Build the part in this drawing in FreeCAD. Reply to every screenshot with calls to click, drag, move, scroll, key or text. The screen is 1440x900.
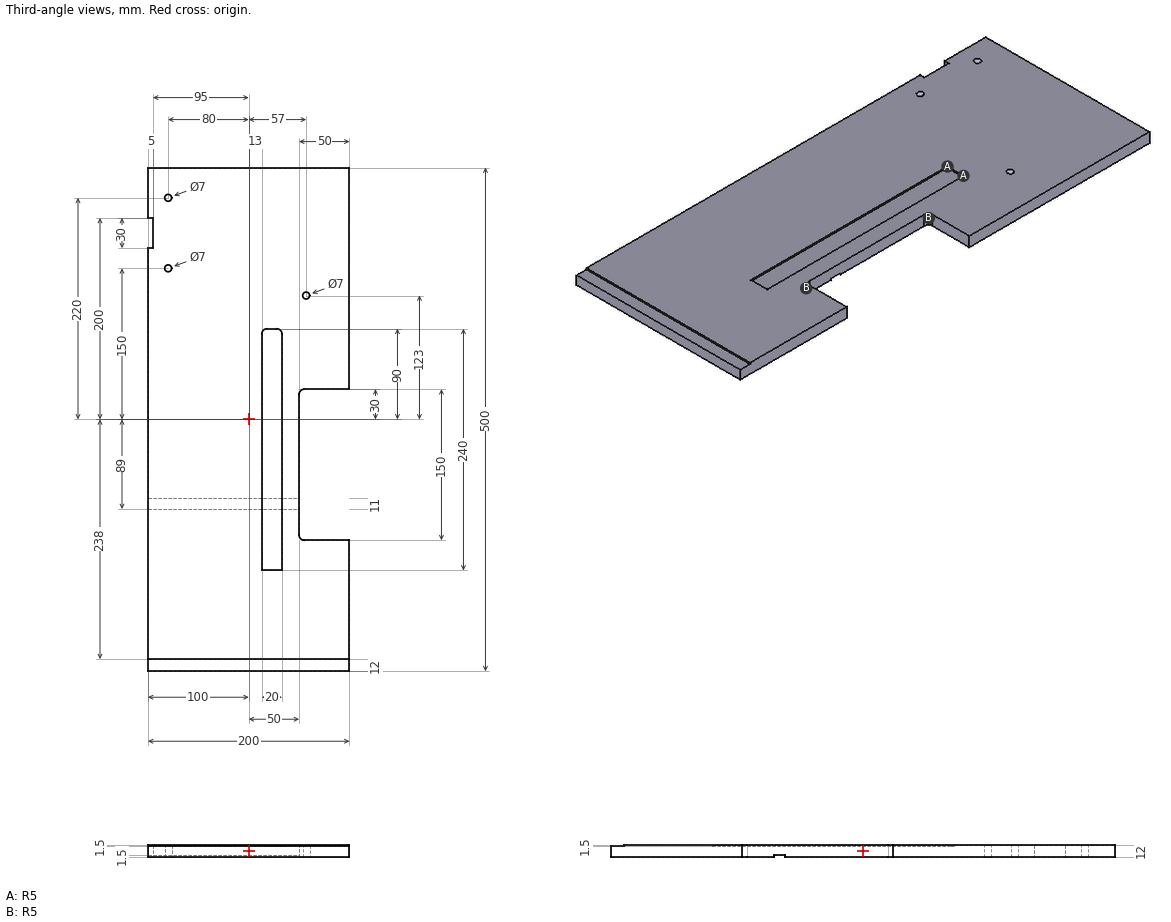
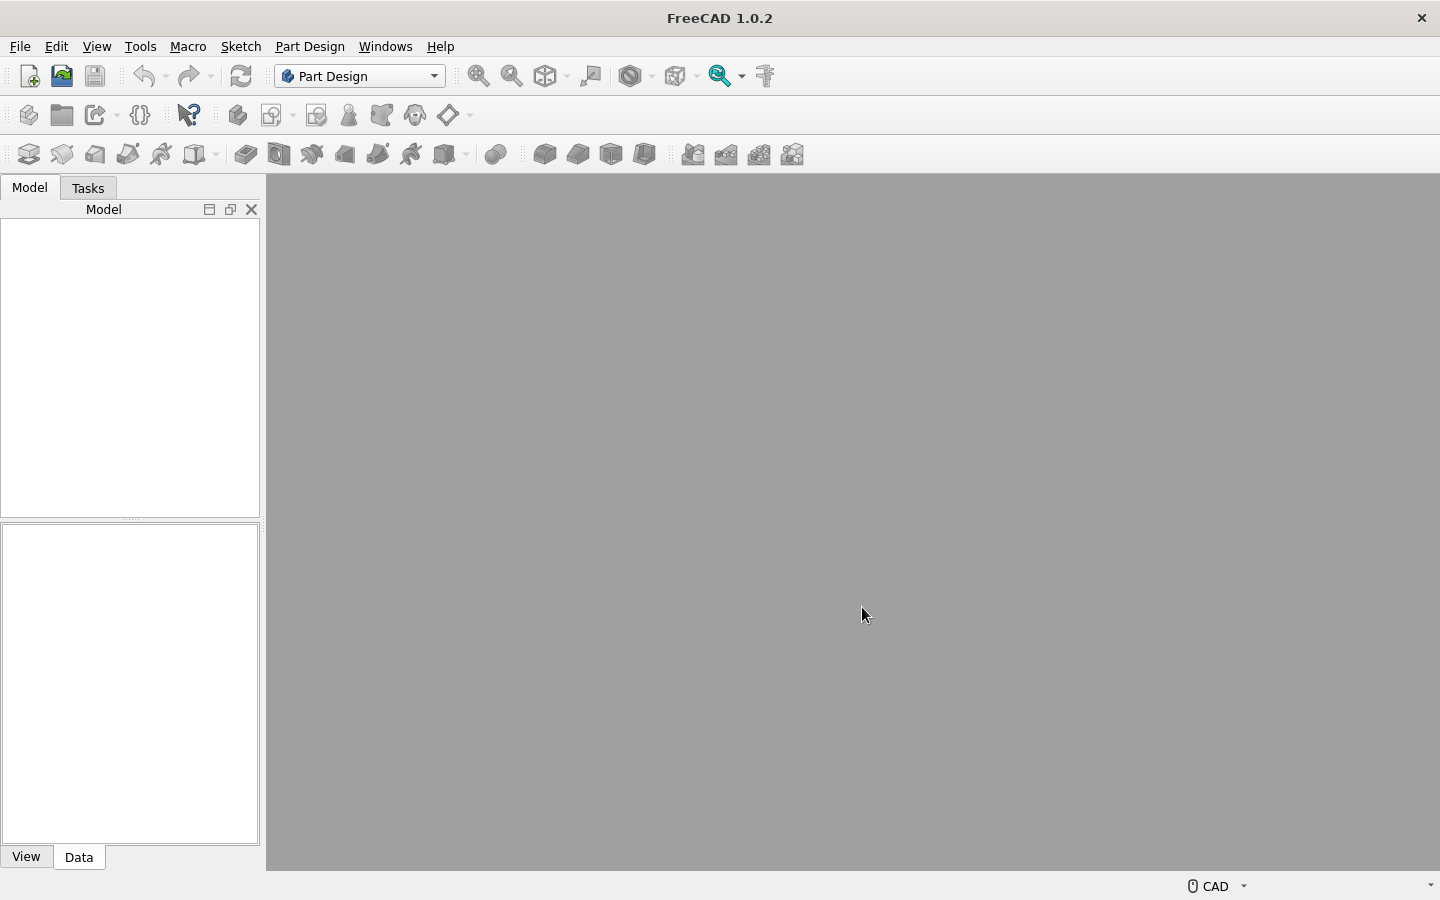
click(29, 76)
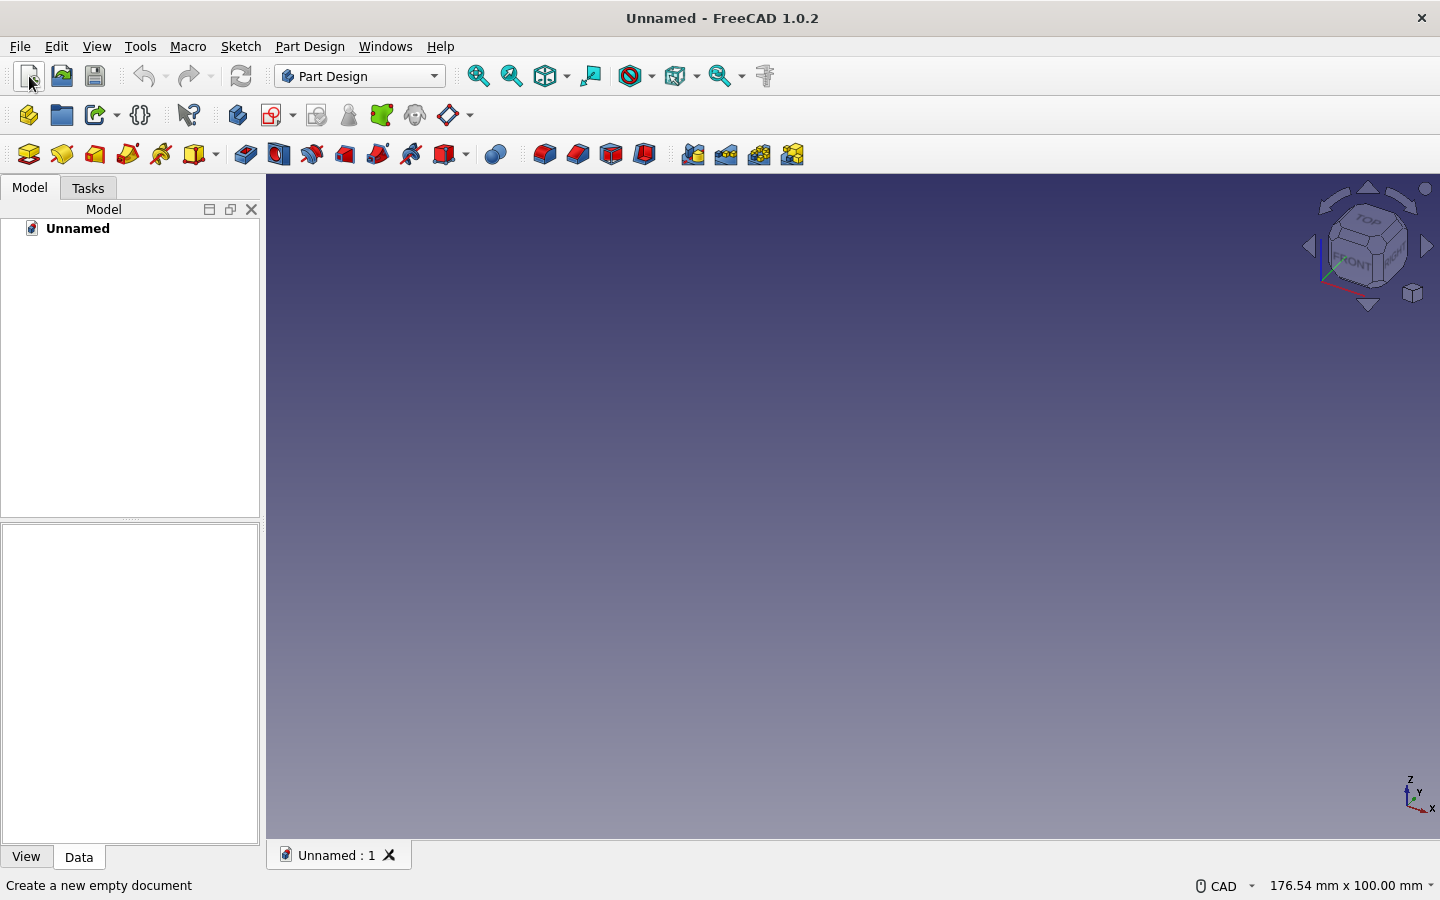
click(270, 116)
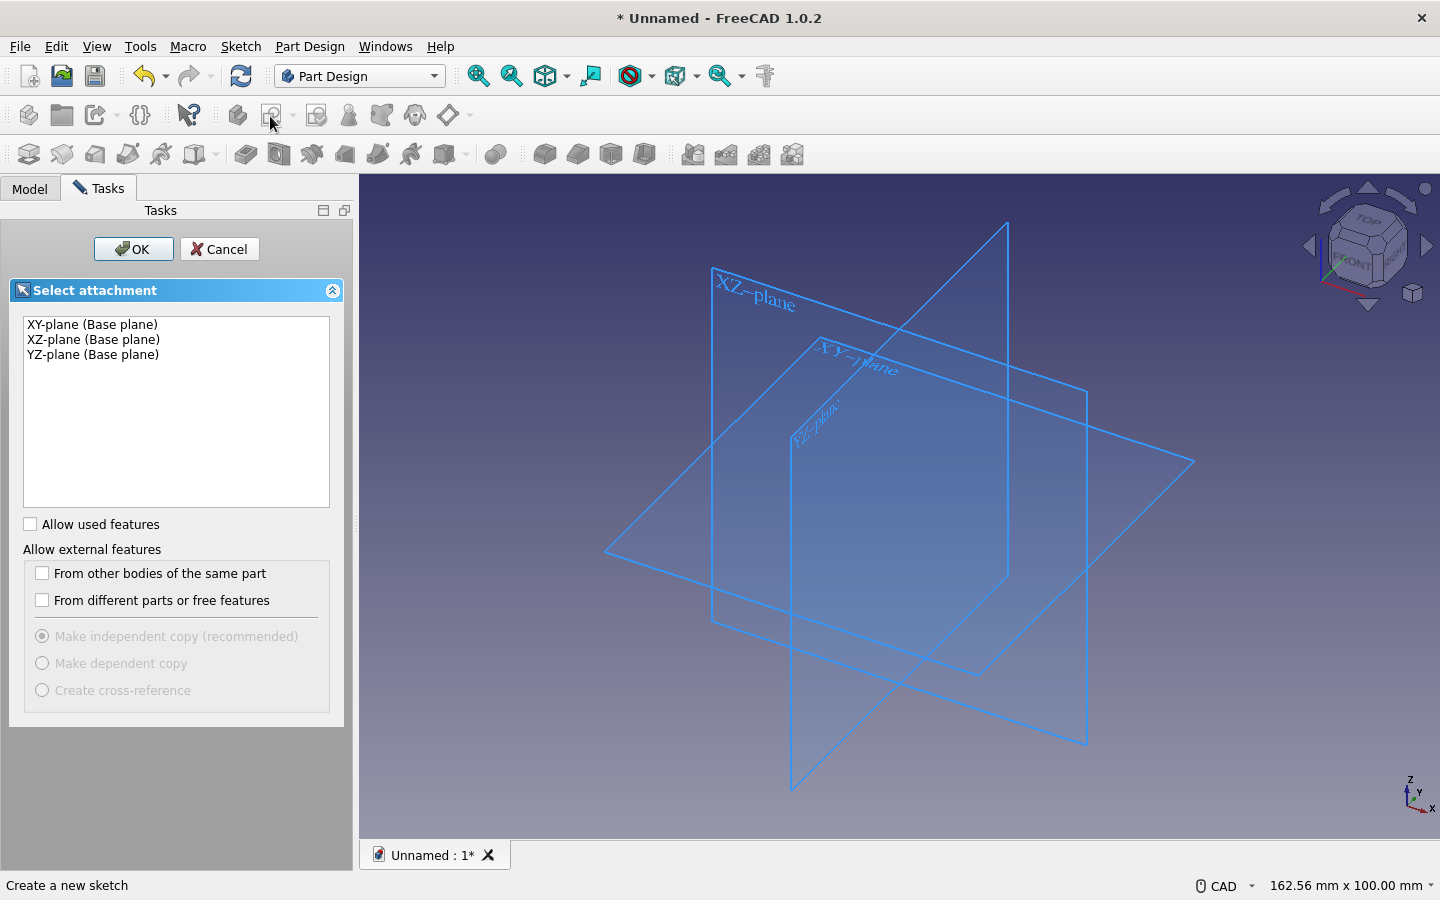
click(84, 324)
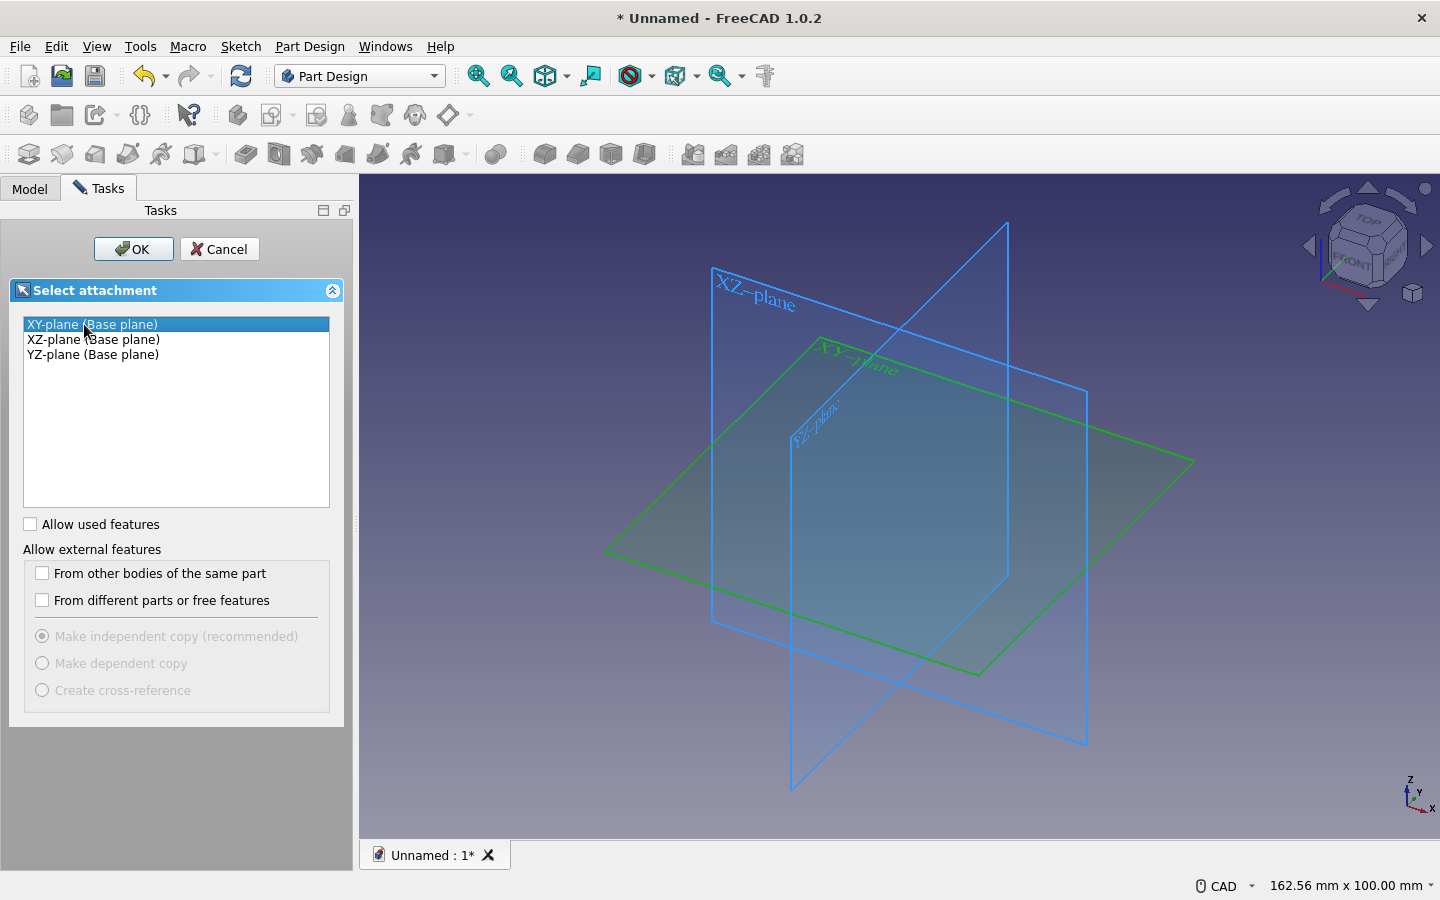
click(134, 249)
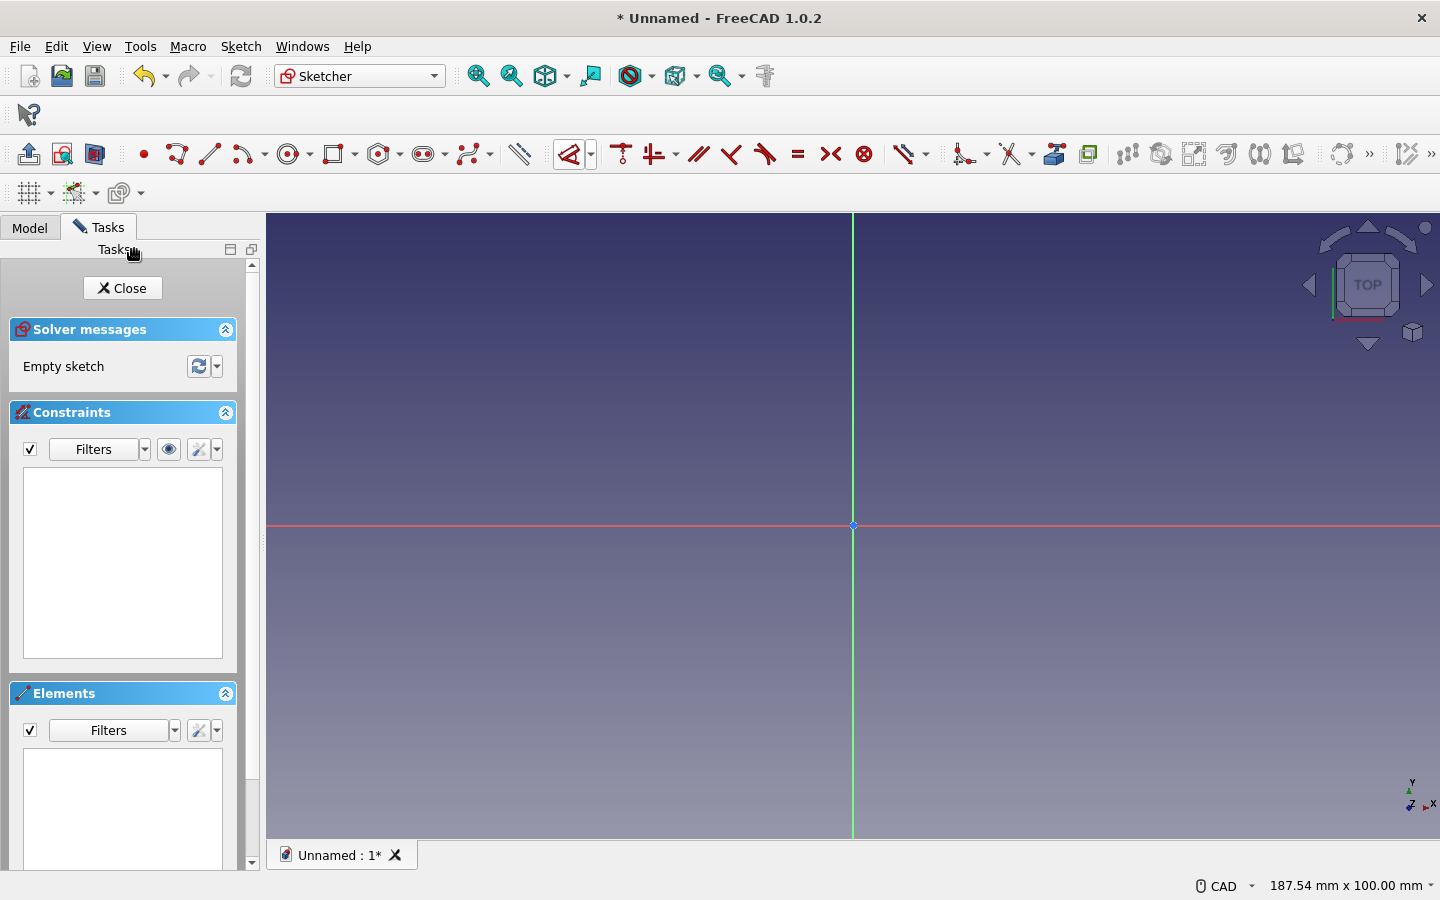
scroll(774, 526, down, 10)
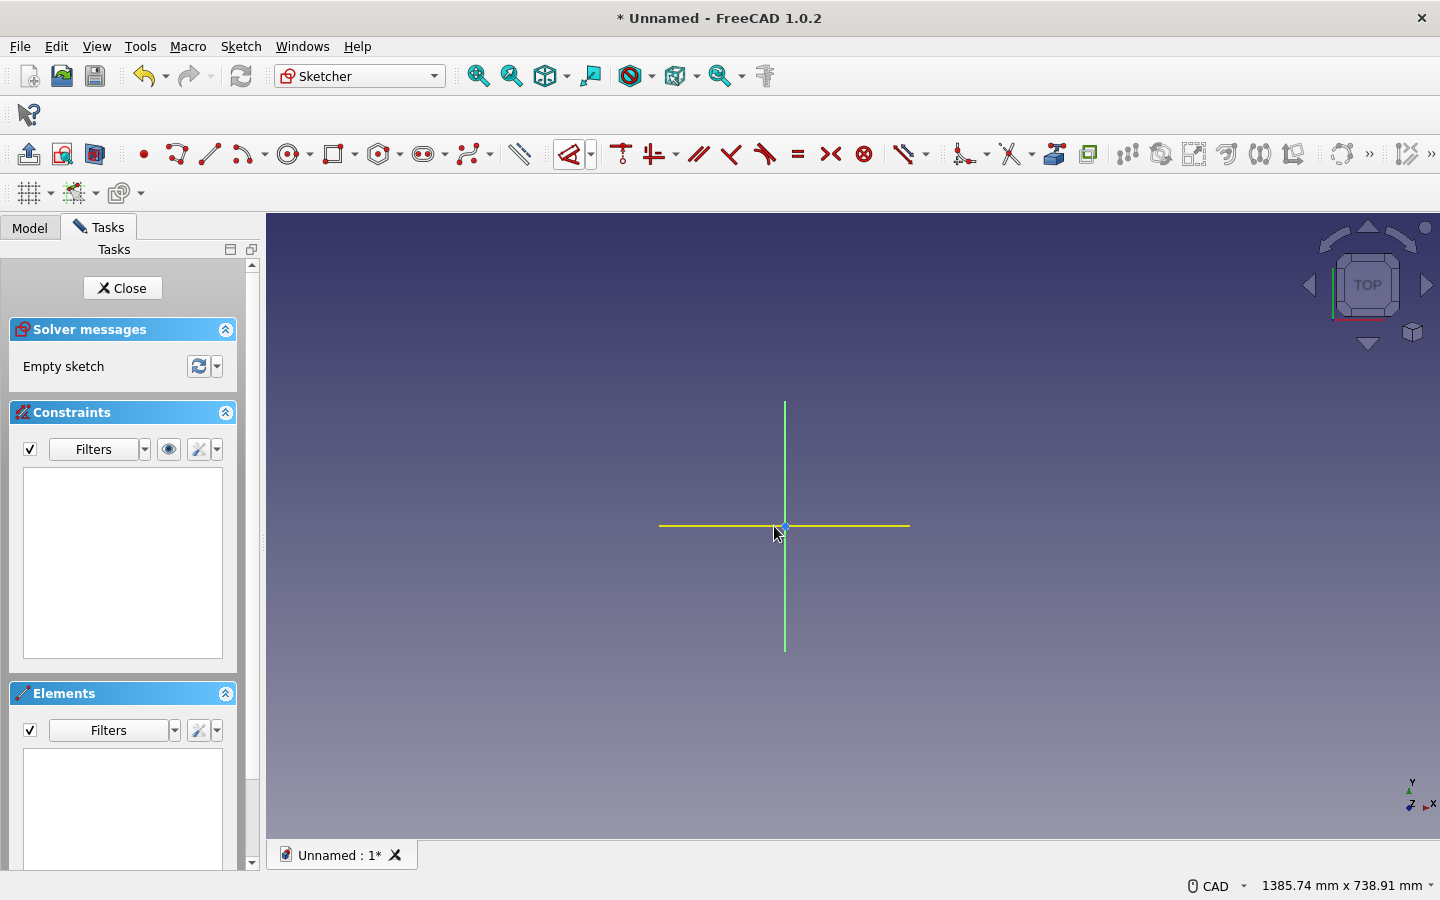
click(354, 154)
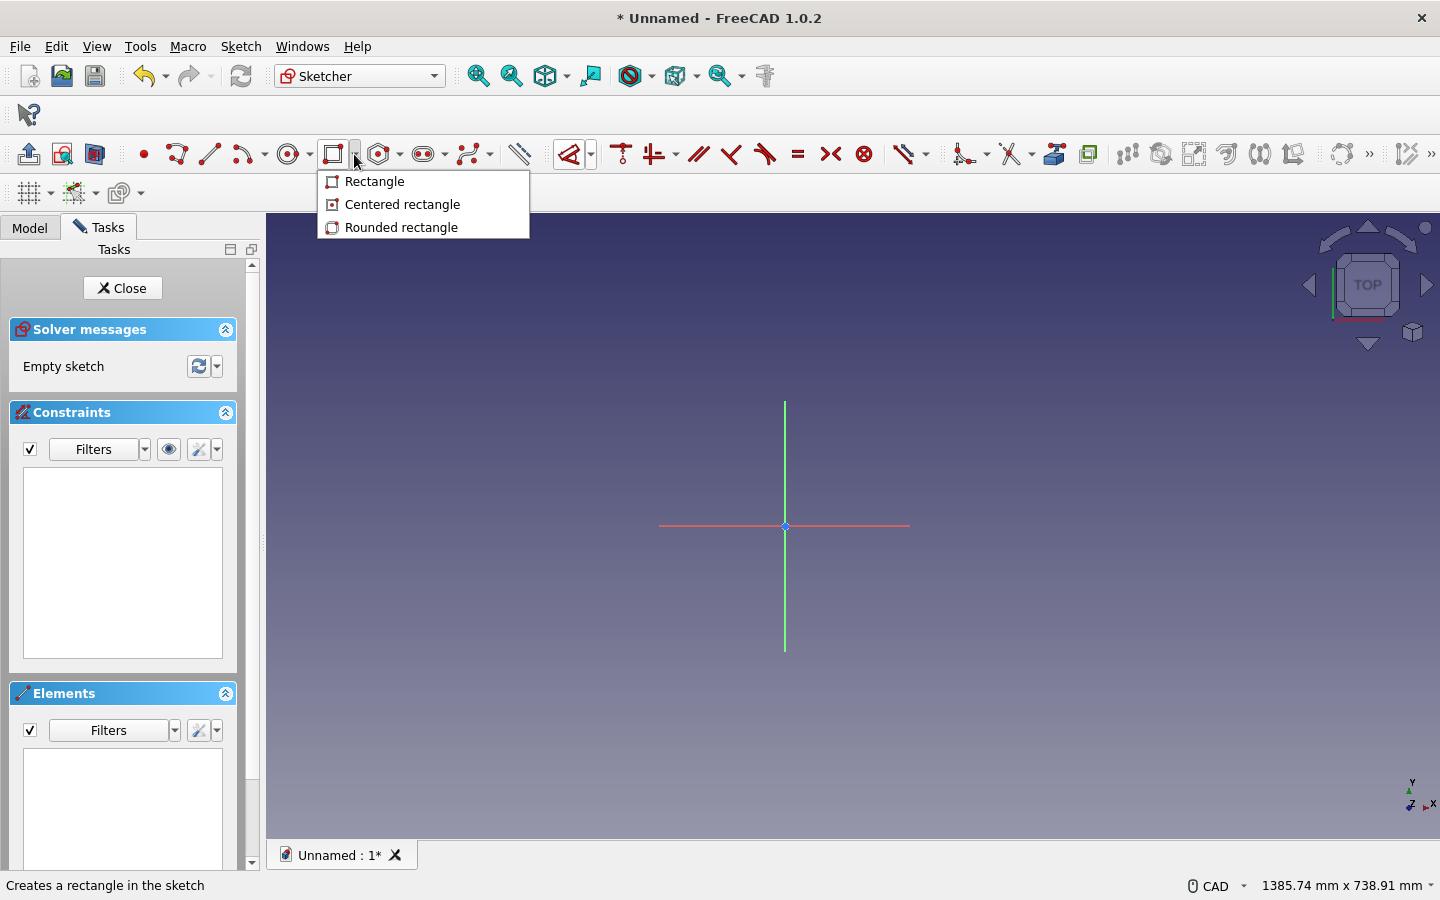
click(424, 204)